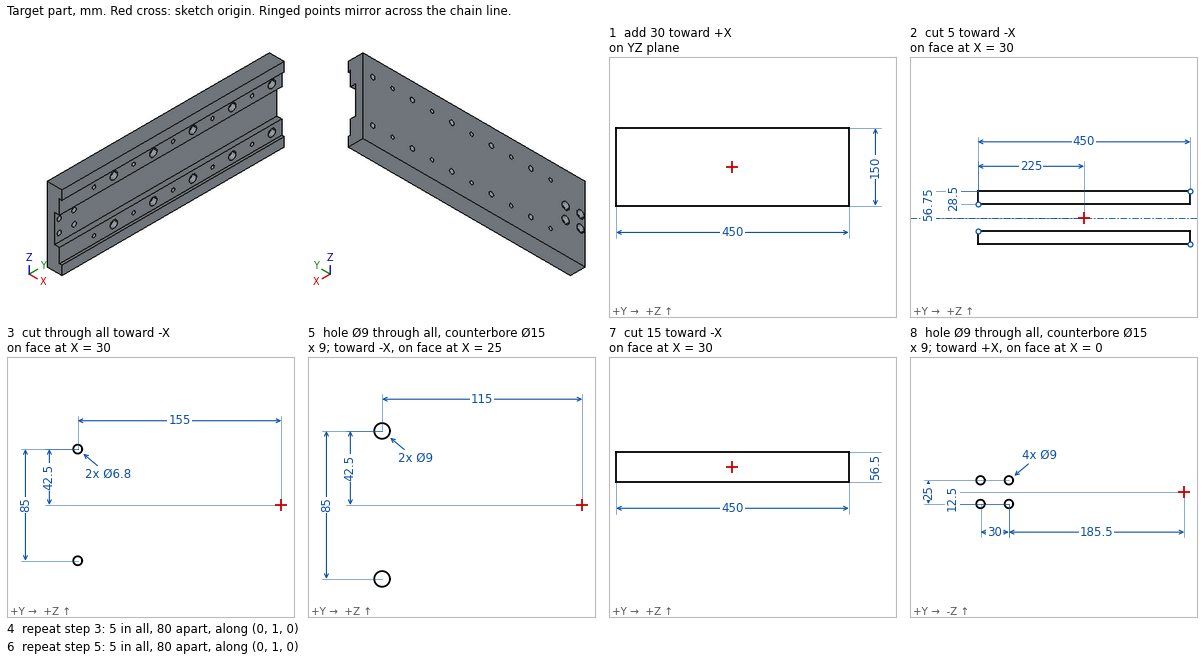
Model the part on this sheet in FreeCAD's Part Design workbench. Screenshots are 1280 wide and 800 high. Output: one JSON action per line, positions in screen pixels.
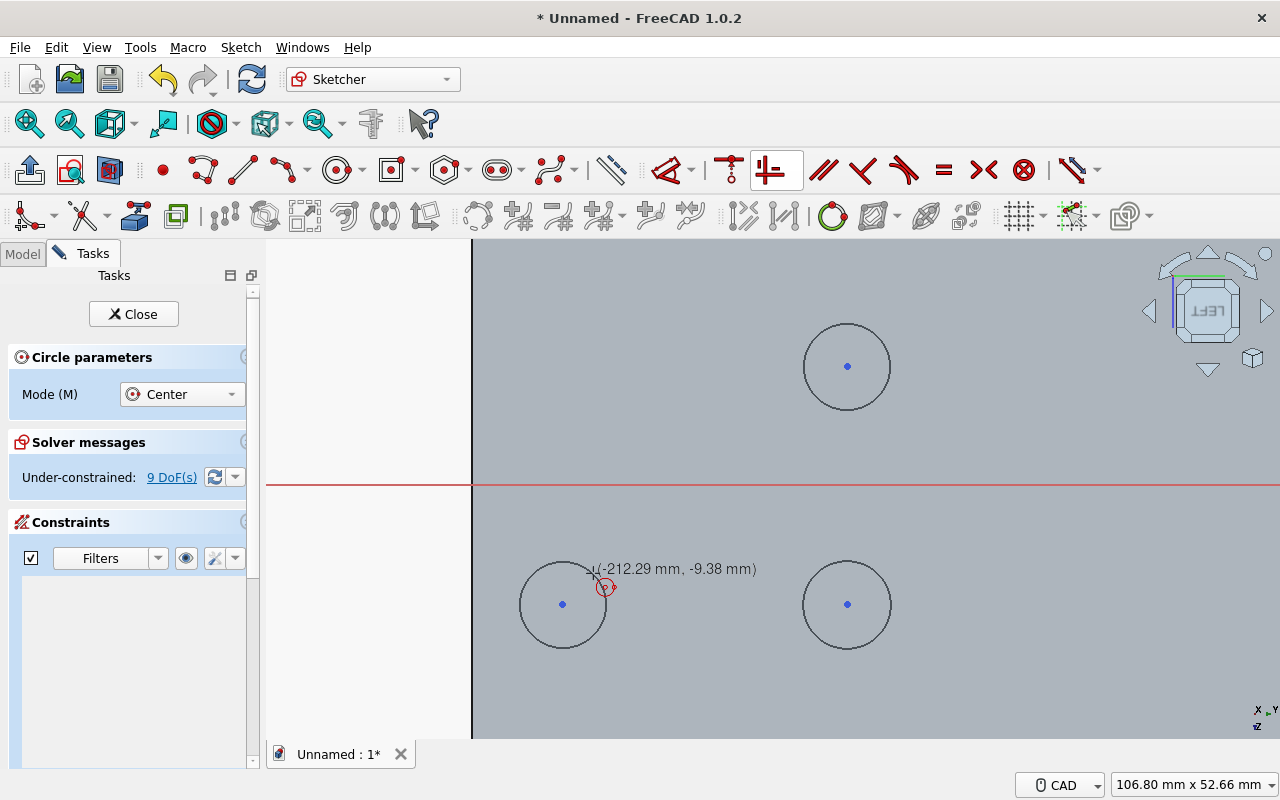
{"action": "left_click", "coordinate": [563, 366]}
{"action": "left_click", "coordinate": [593, 336]}
{"action": "key", "text": "Escape"}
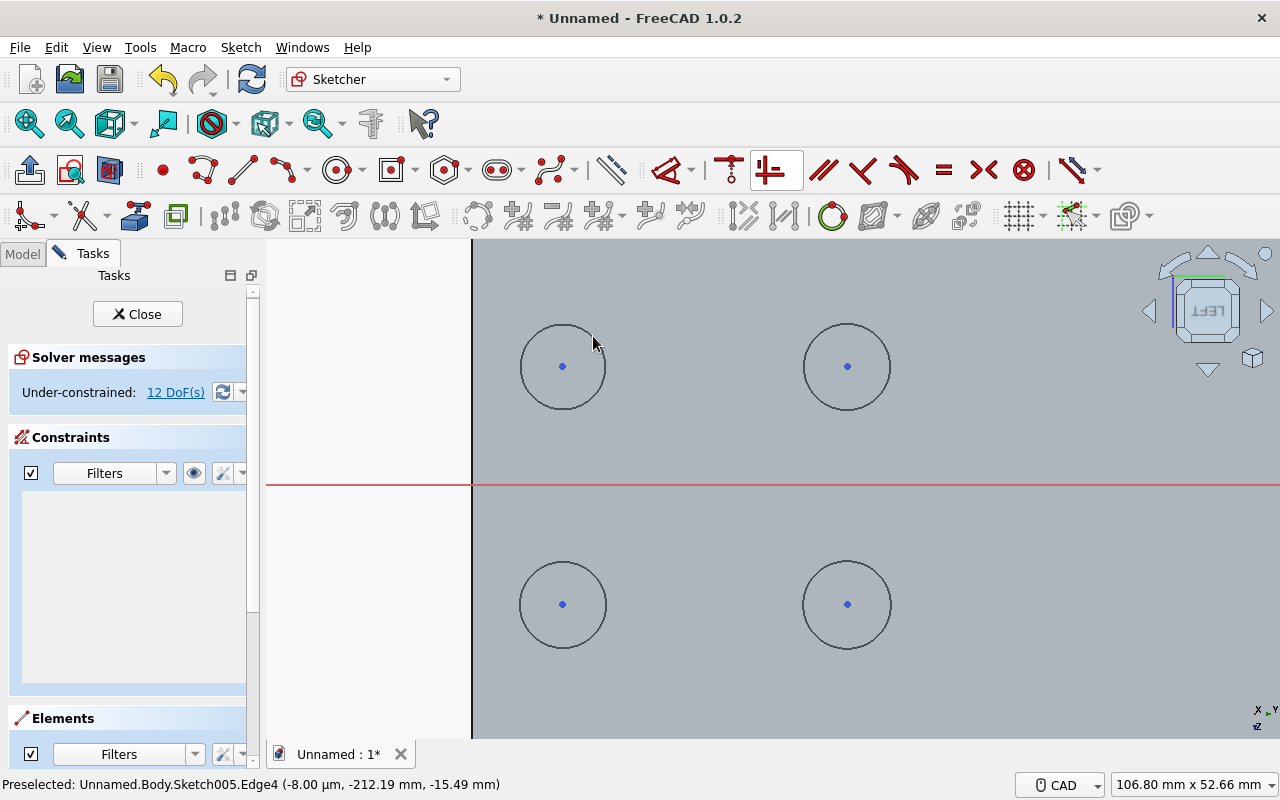
{"action": "left_click", "coordinate": [878, 574]}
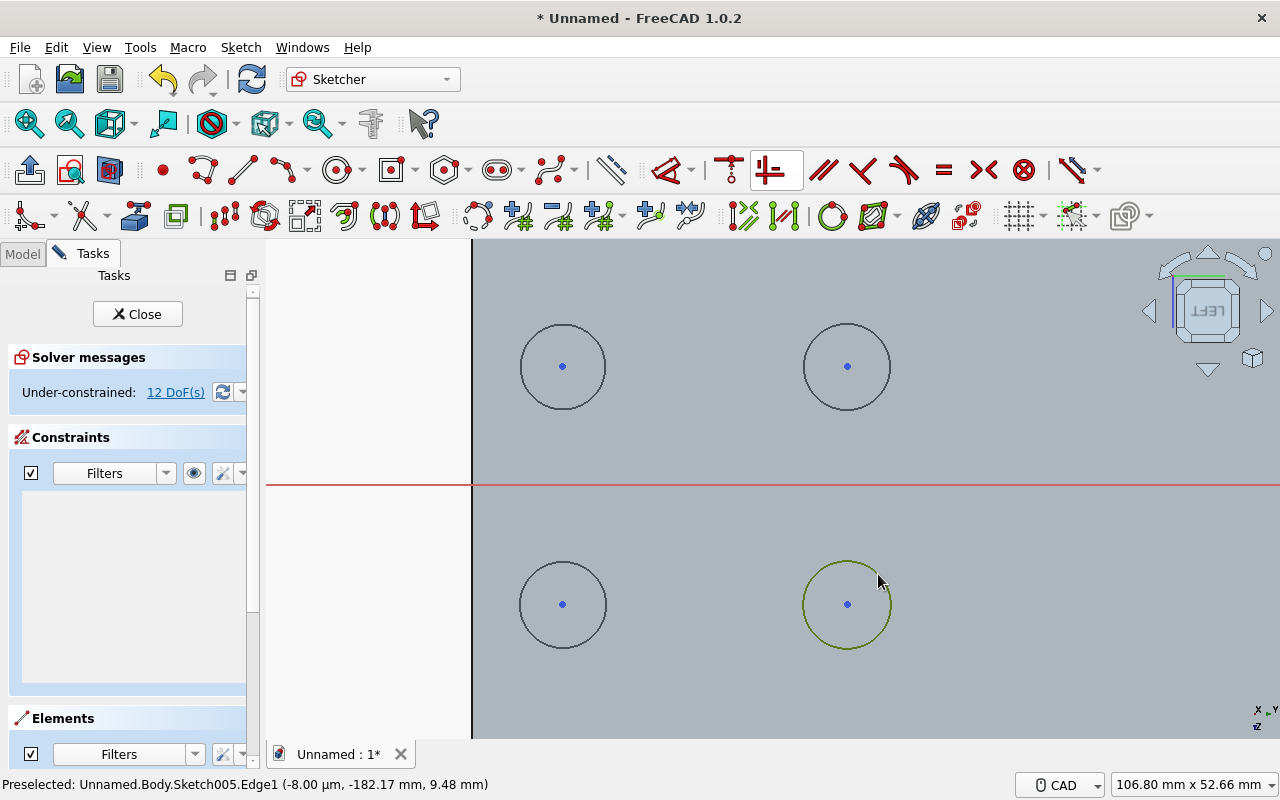
{"action": "left_click", "coordinate": [877, 336]}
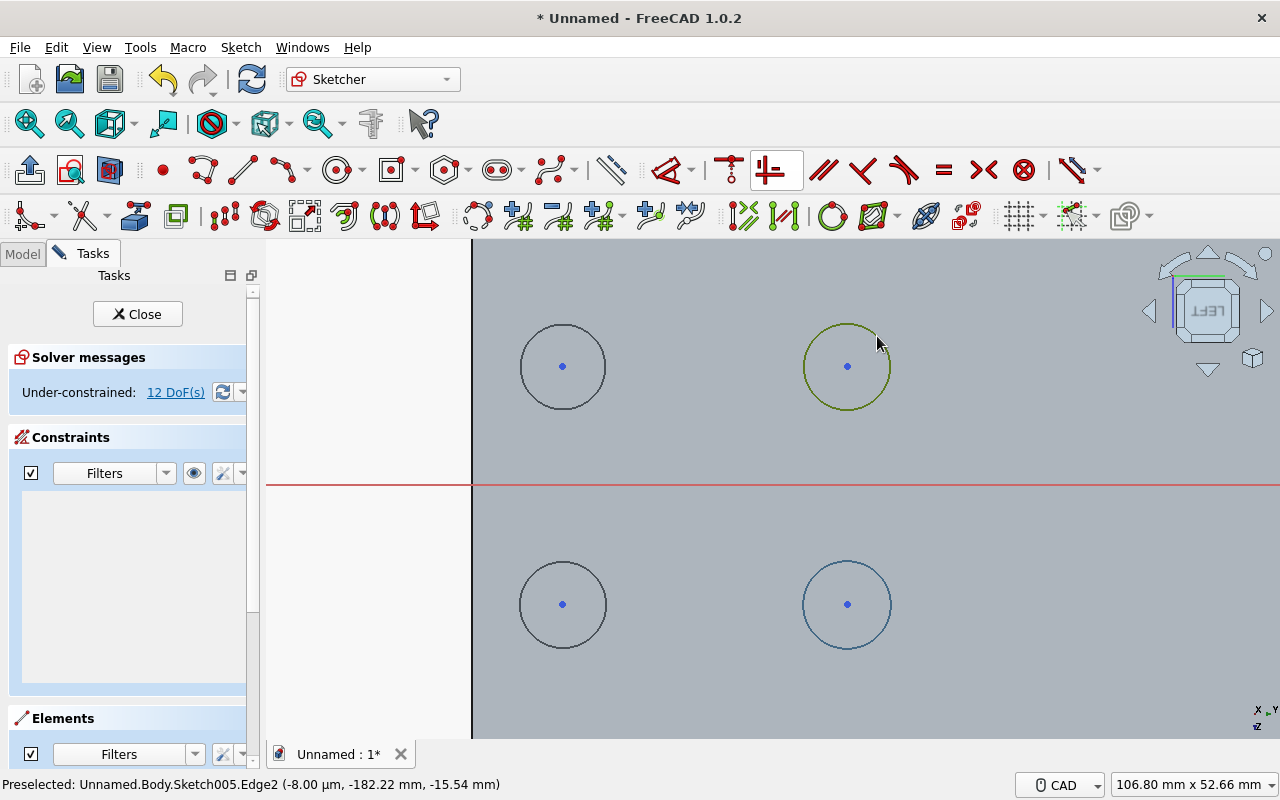
{"action": "left_click", "coordinate": [593, 574]}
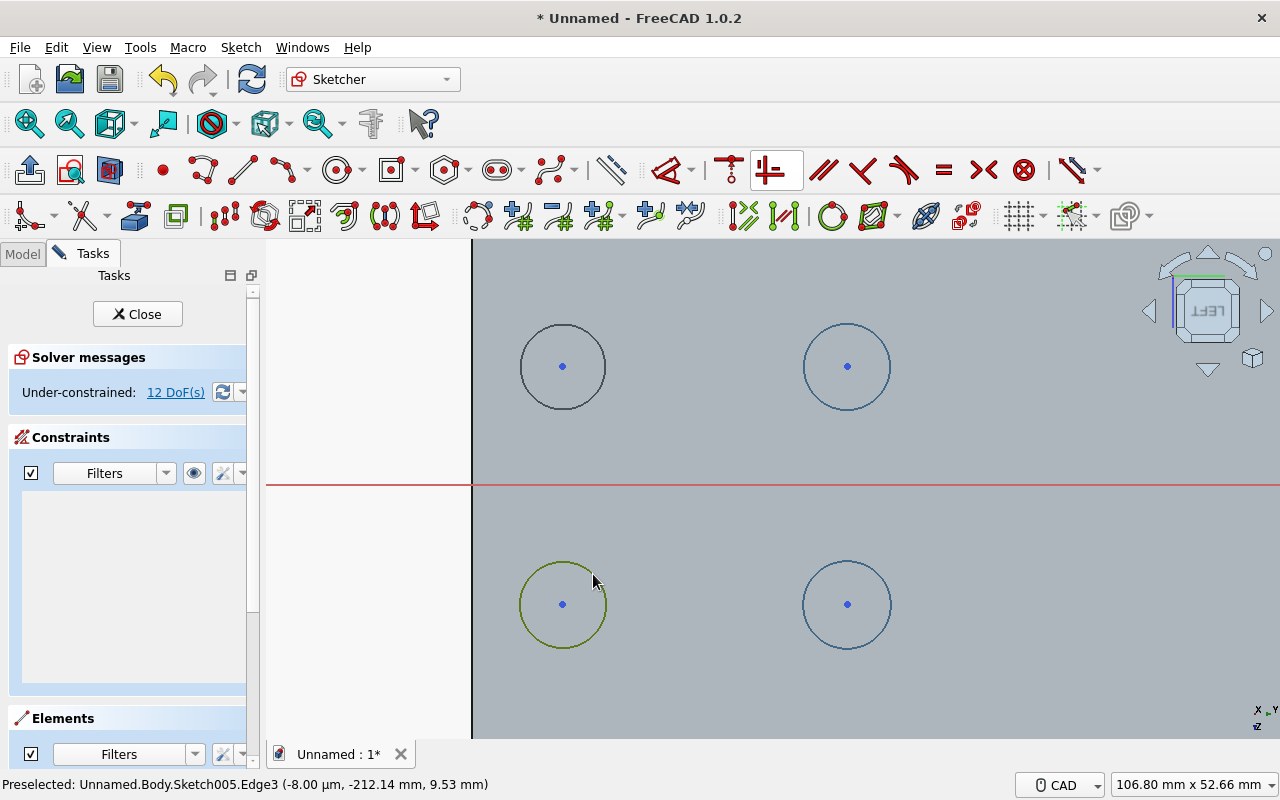
{"action": "left_click", "coordinate": [593, 337]}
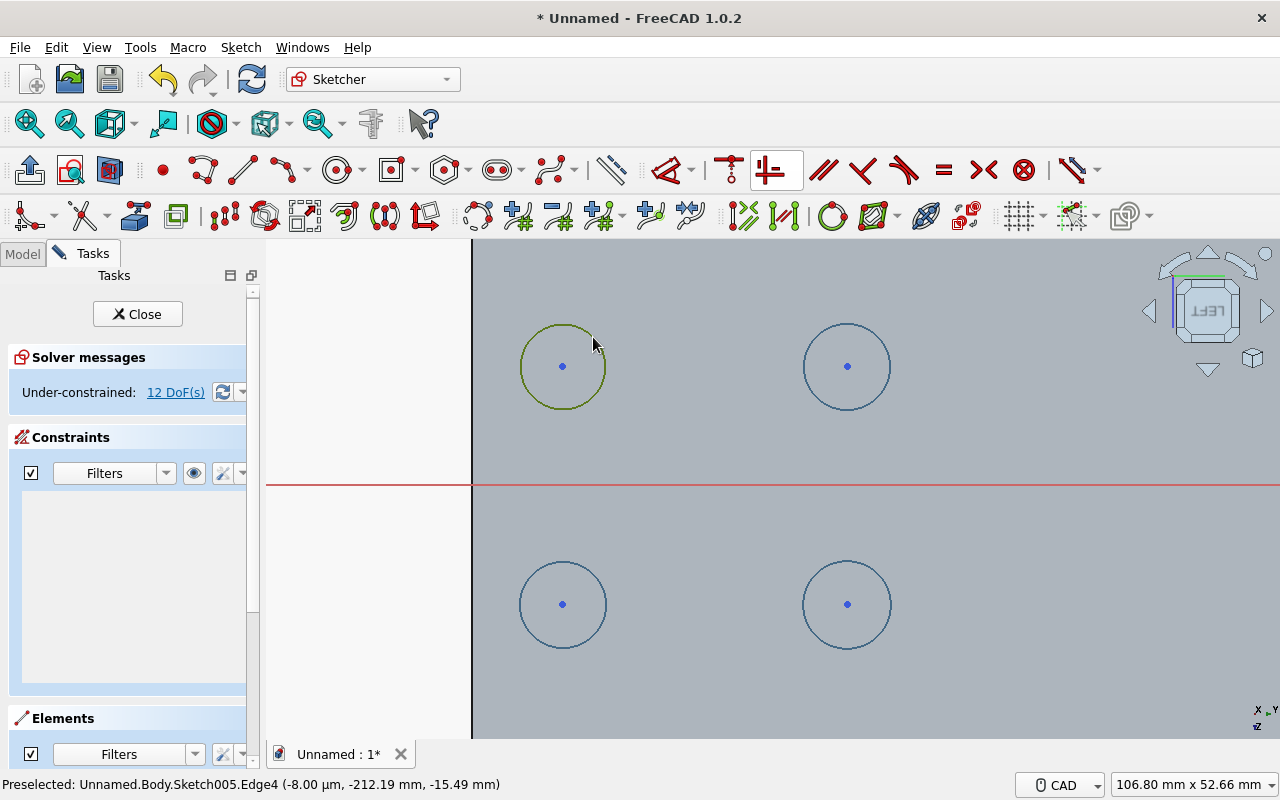
{"action": "left_click", "coordinate": [944, 170]}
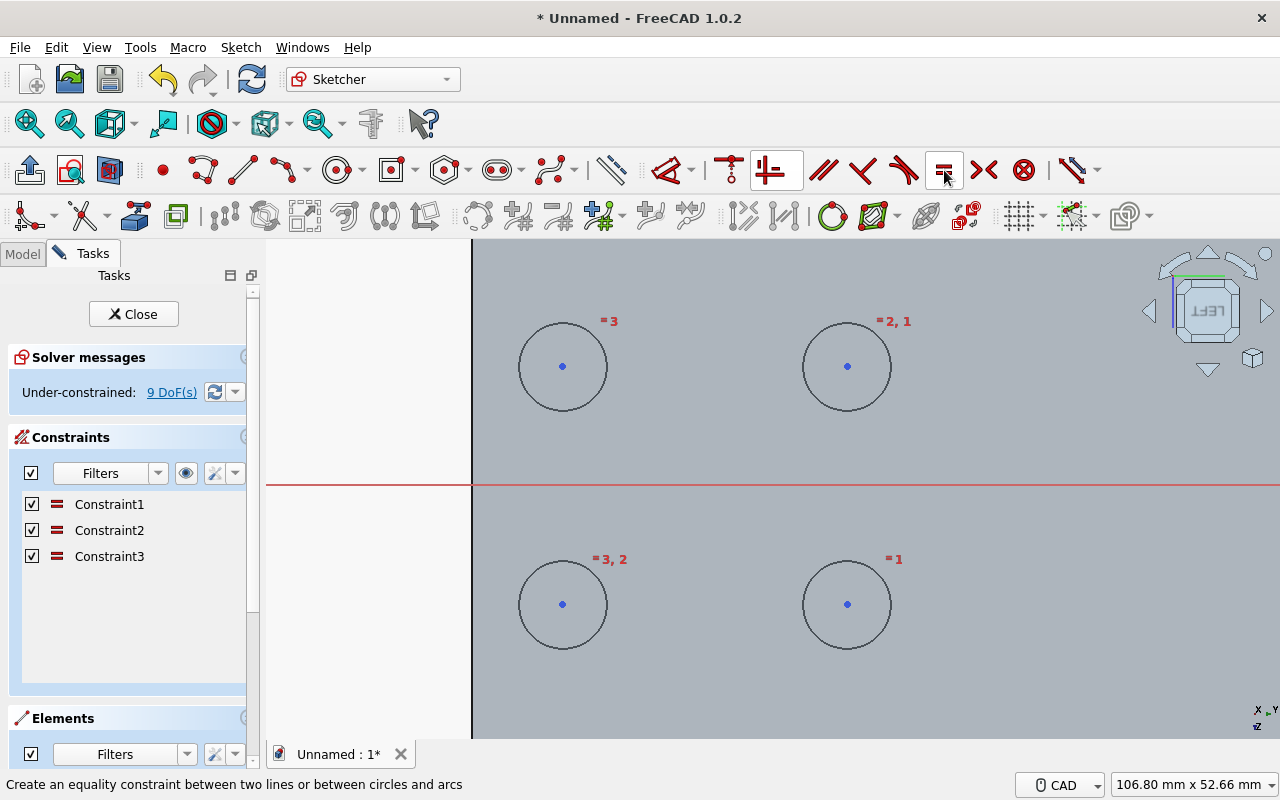
{"action": "left_click", "coordinate": [847, 605]}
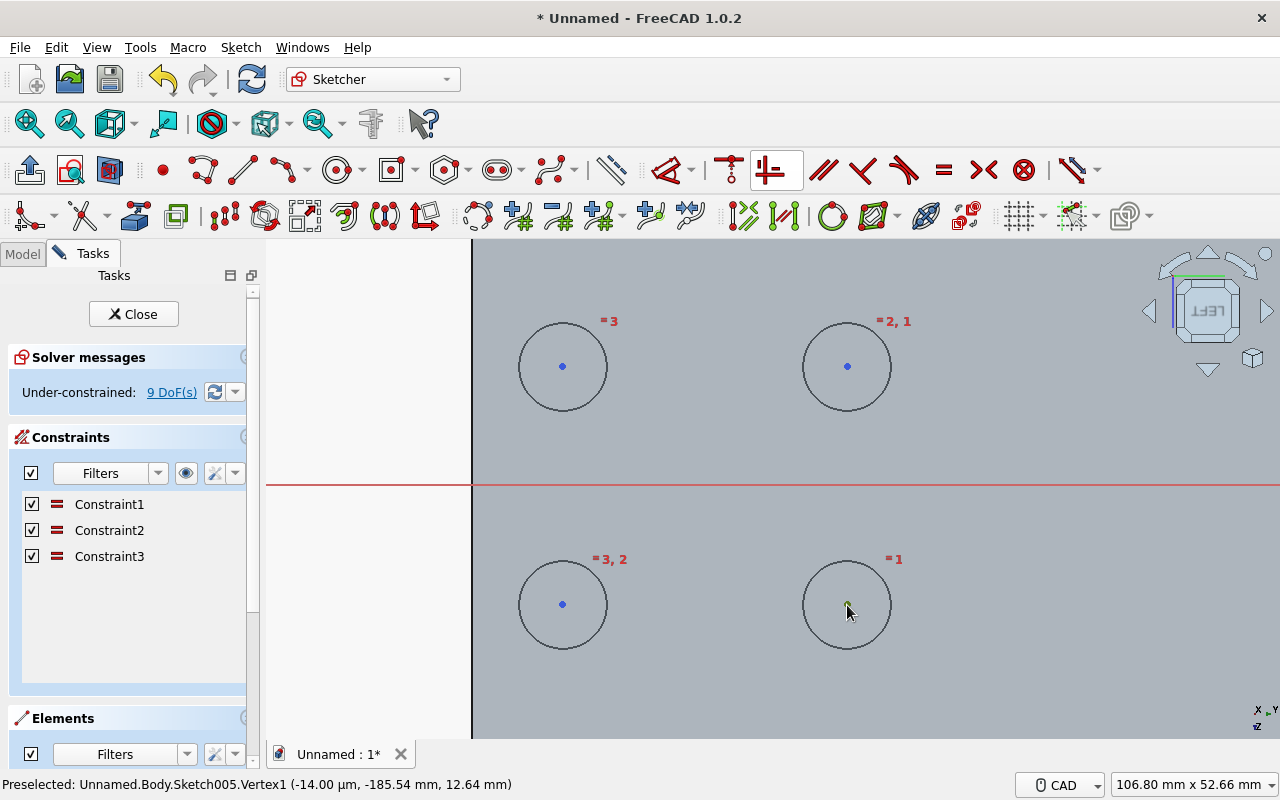
{"action": "left_click", "coordinate": [847, 367]}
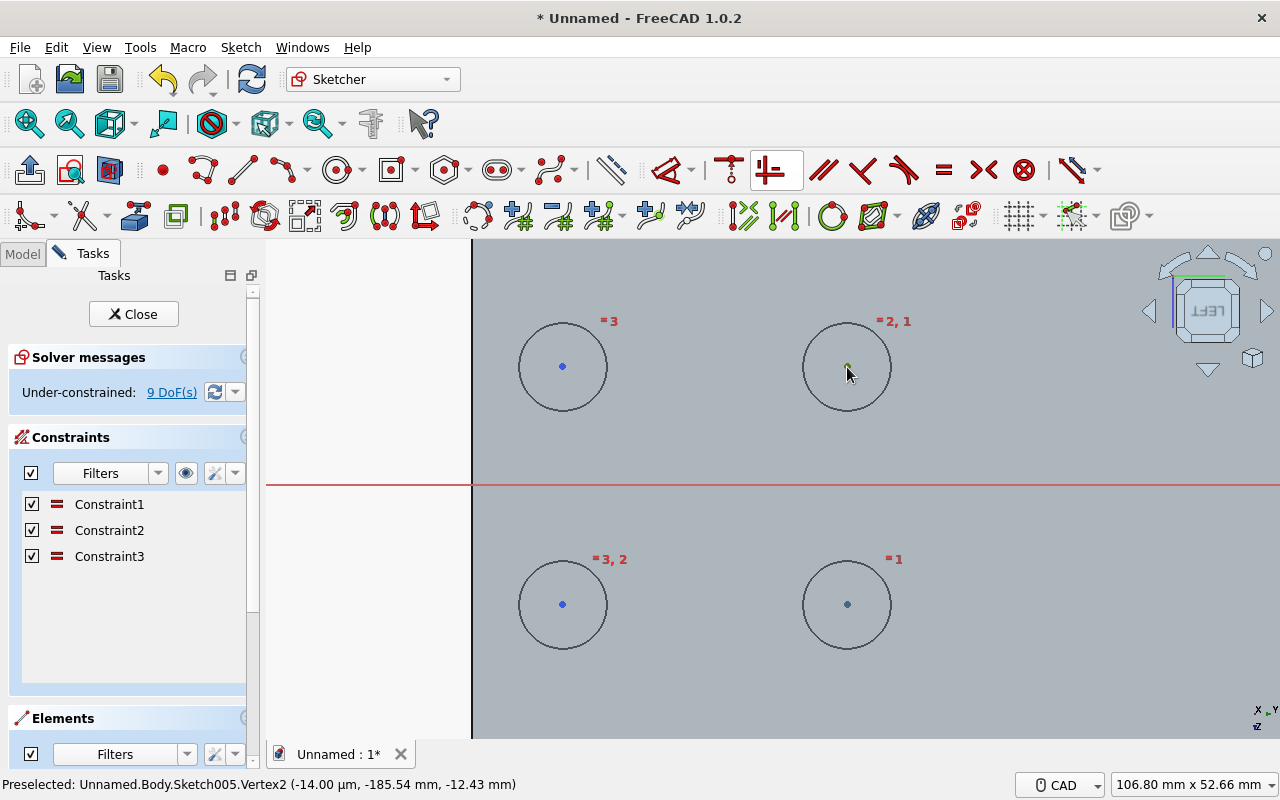
{"action": "key", "text": "v"}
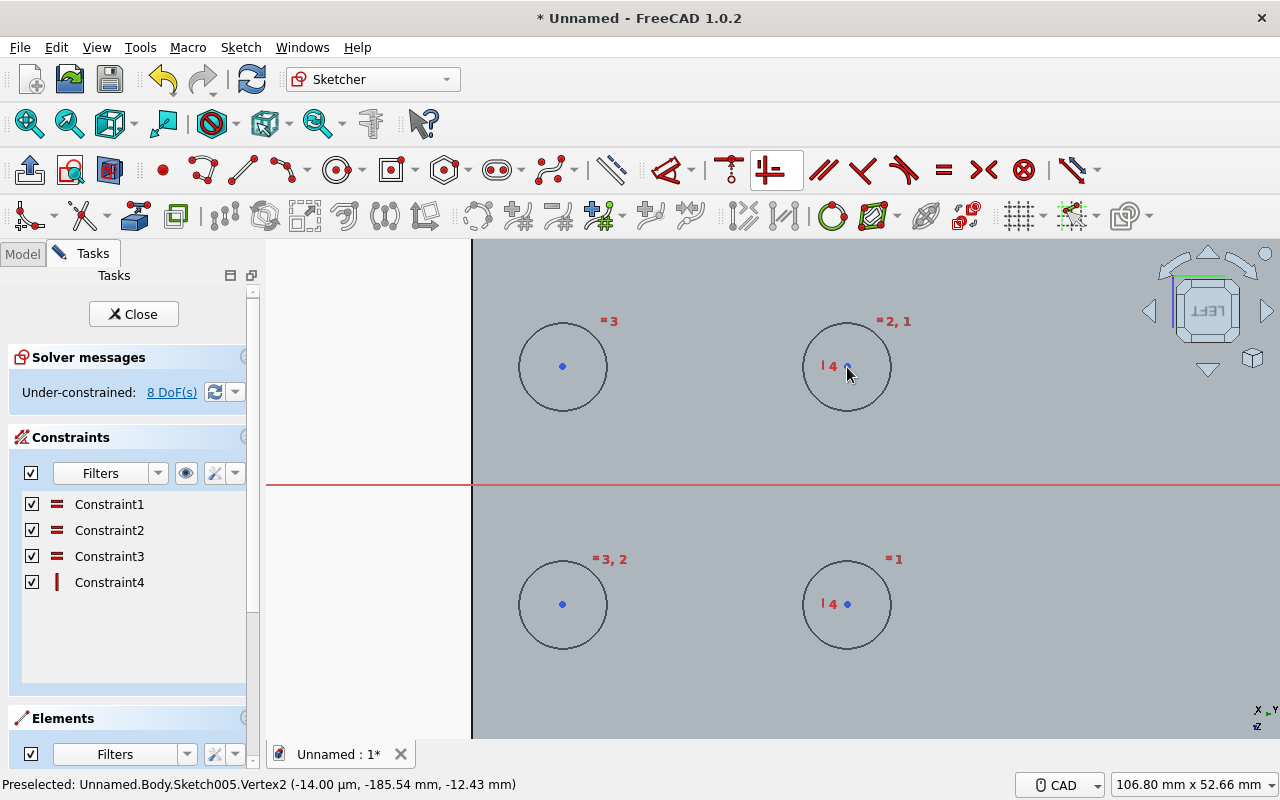
{"action": "left_click", "coordinate": [847, 605]}